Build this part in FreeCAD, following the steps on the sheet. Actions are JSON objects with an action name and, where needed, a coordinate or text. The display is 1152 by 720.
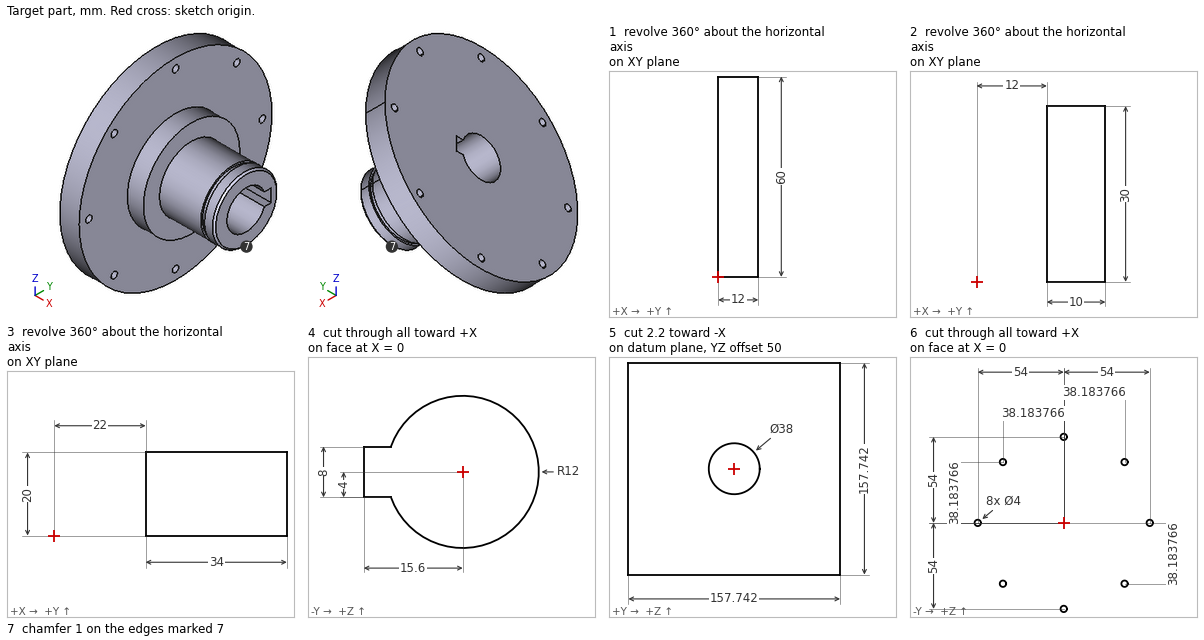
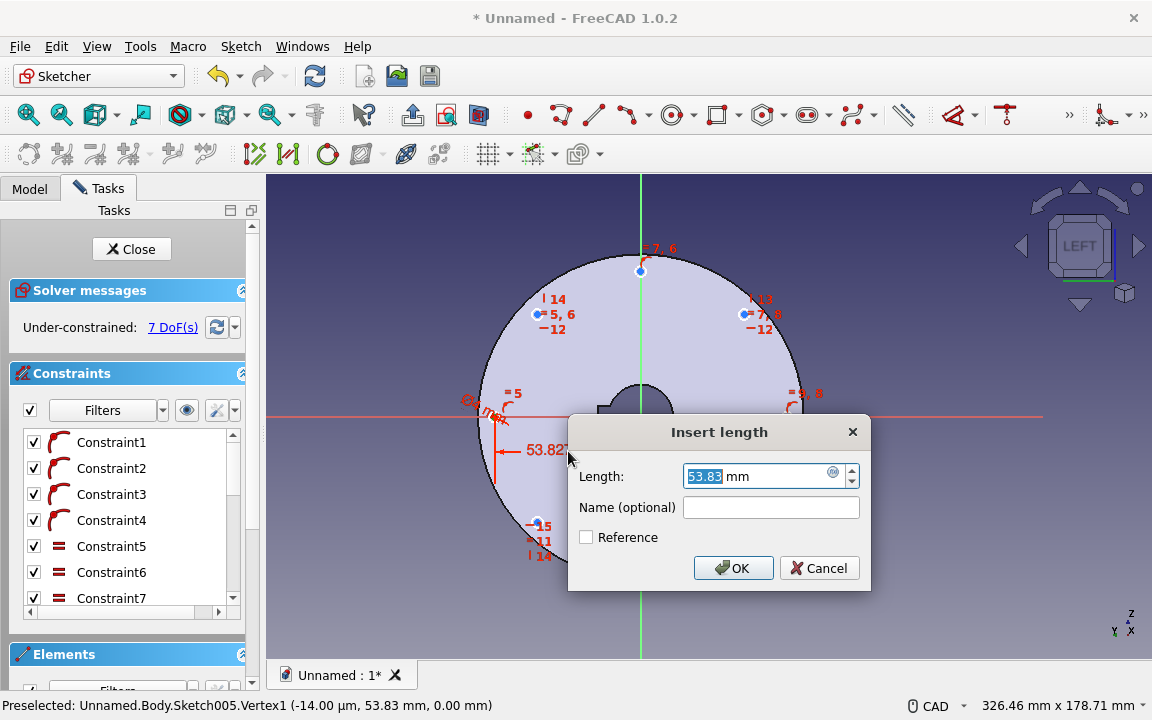
{"action": "type", "text": "54"}
{"action": "key", "text": "Return"}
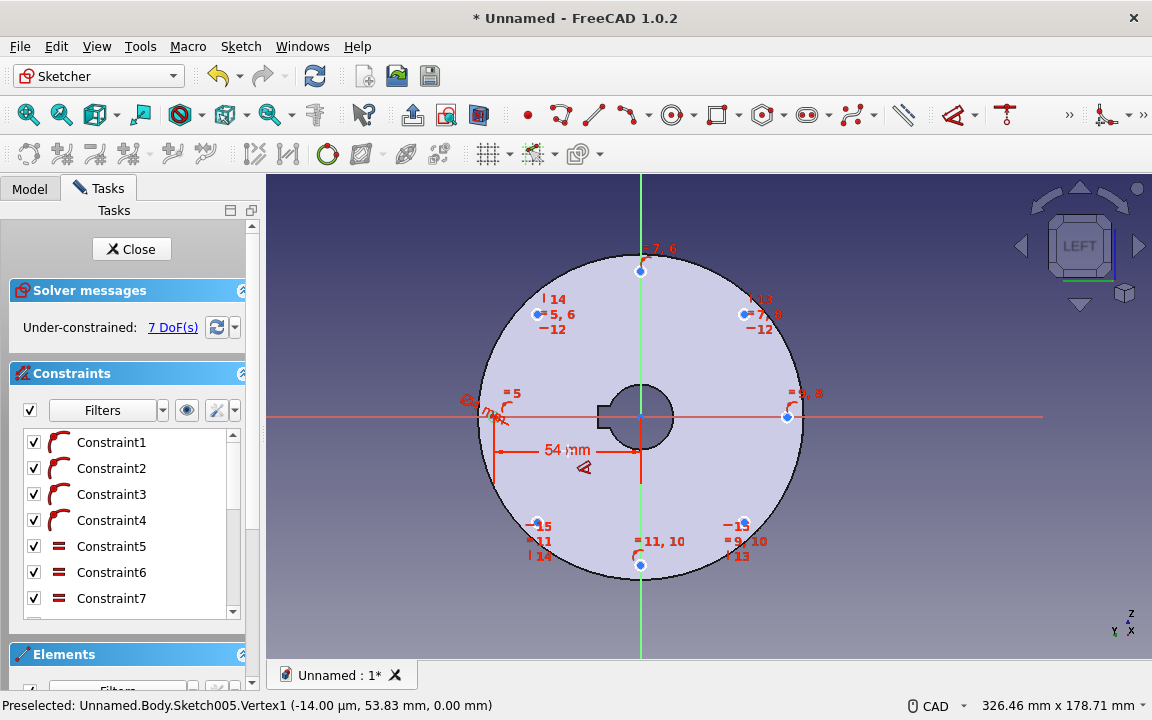
{"action": "left_click", "coordinate": [641, 272]}
{"action": "left_click", "coordinate": [675, 344]}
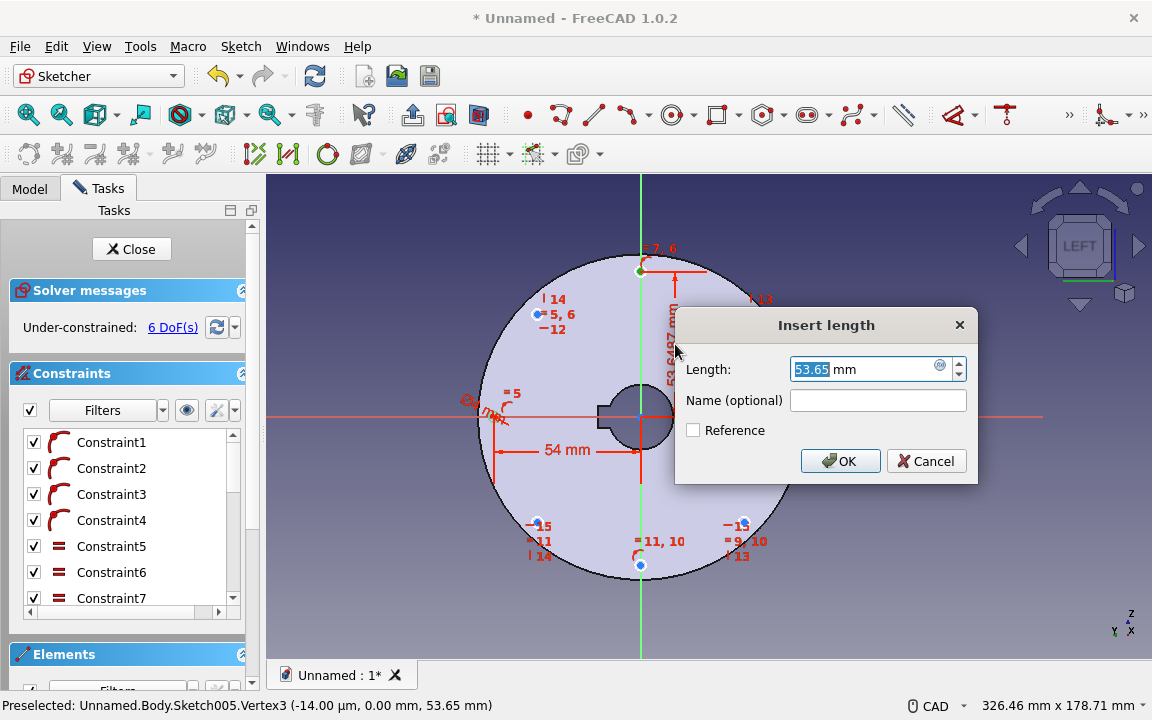
{"action": "type", "text": "54"}
{"action": "key", "text": "Return"}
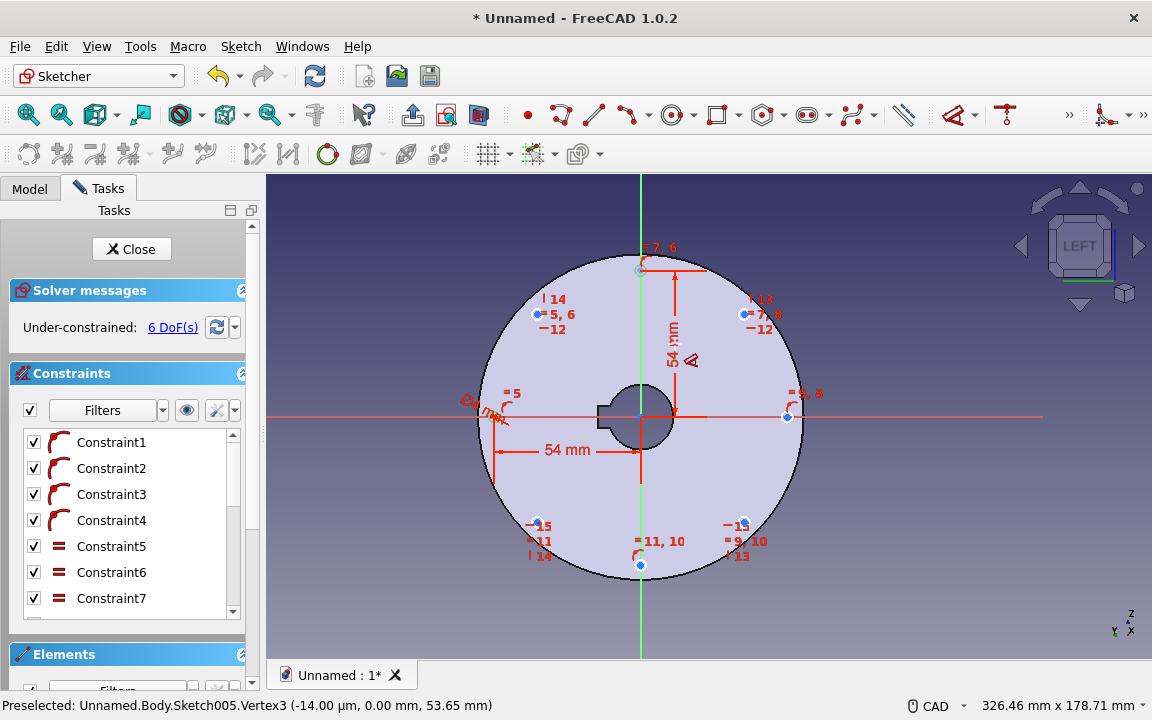
{"action": "left_click", "coordinate": [787, 417]}
{"action": "left_click", "coordinate": [714, 451]}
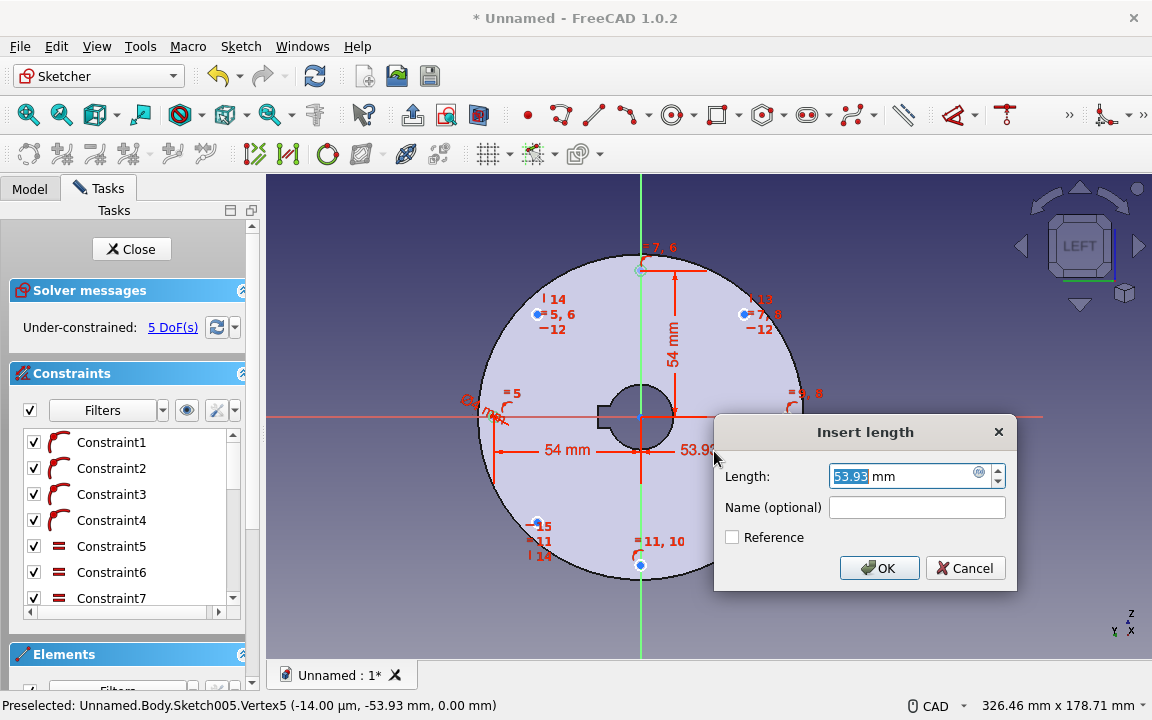
{"action": "type", "text": "54"}
{"action": "key", "text": "Return"}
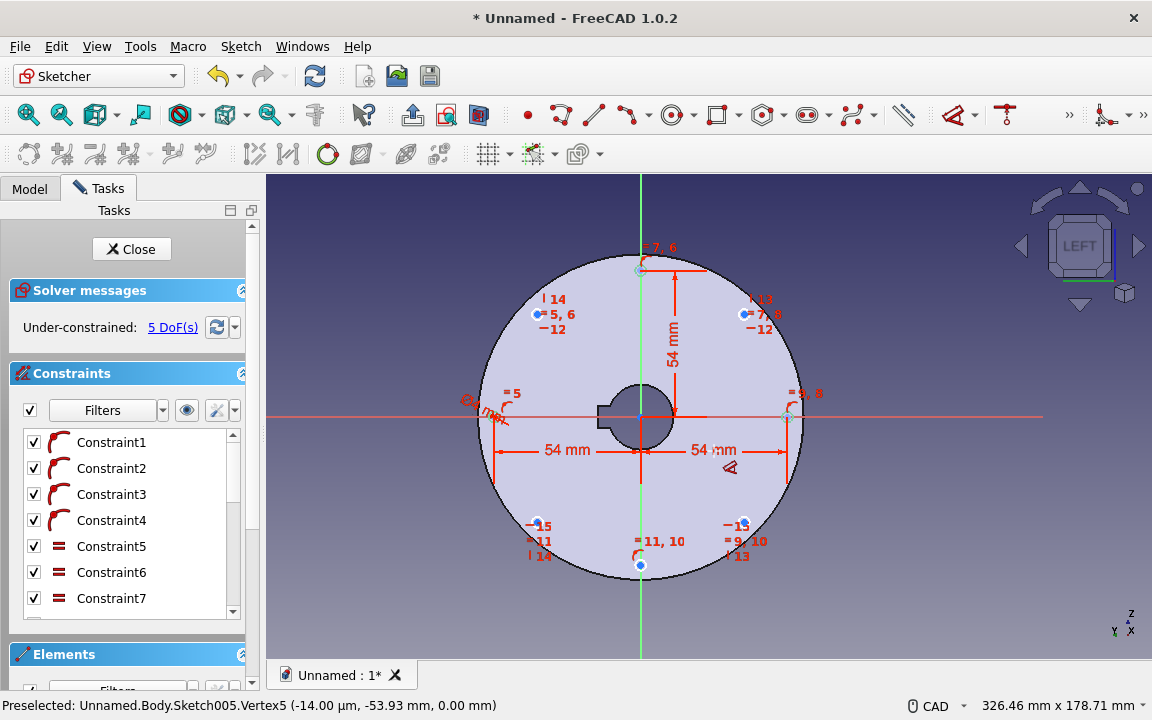
{"action": "left_click", "coordinate": [641, 565]}
{"action": "left_click", "coordinate": [675, 491]}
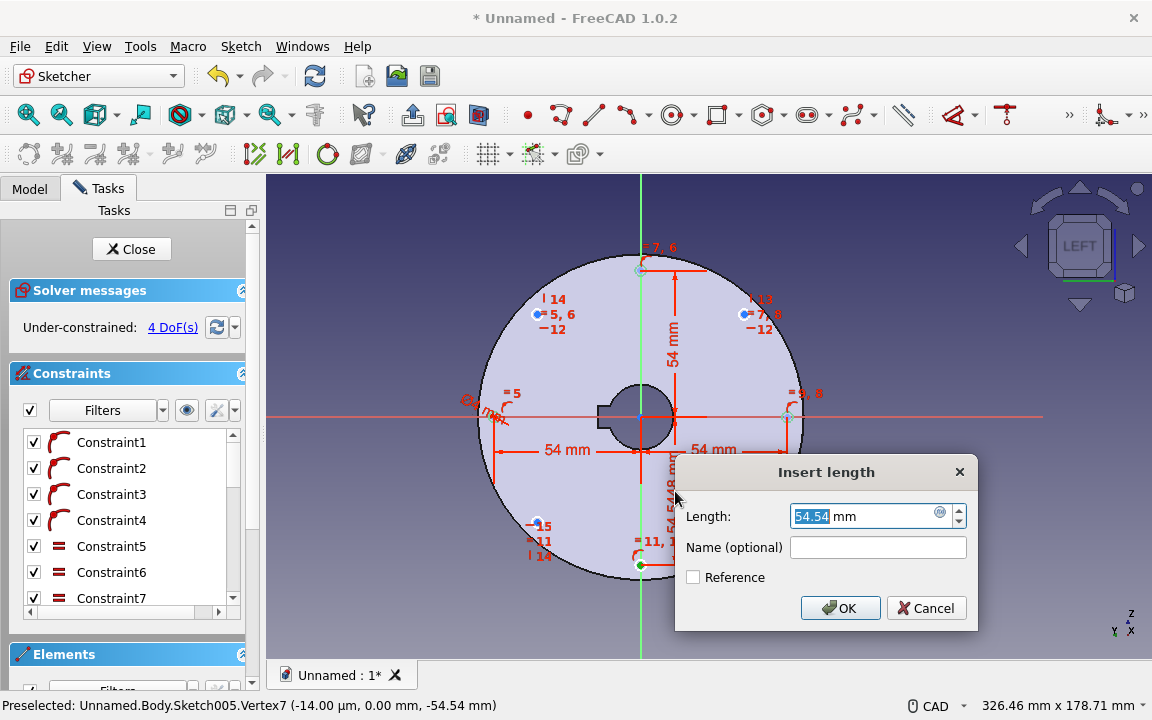
{"action": "type", "text": "54"}
{"action": "key", "text": "Return"}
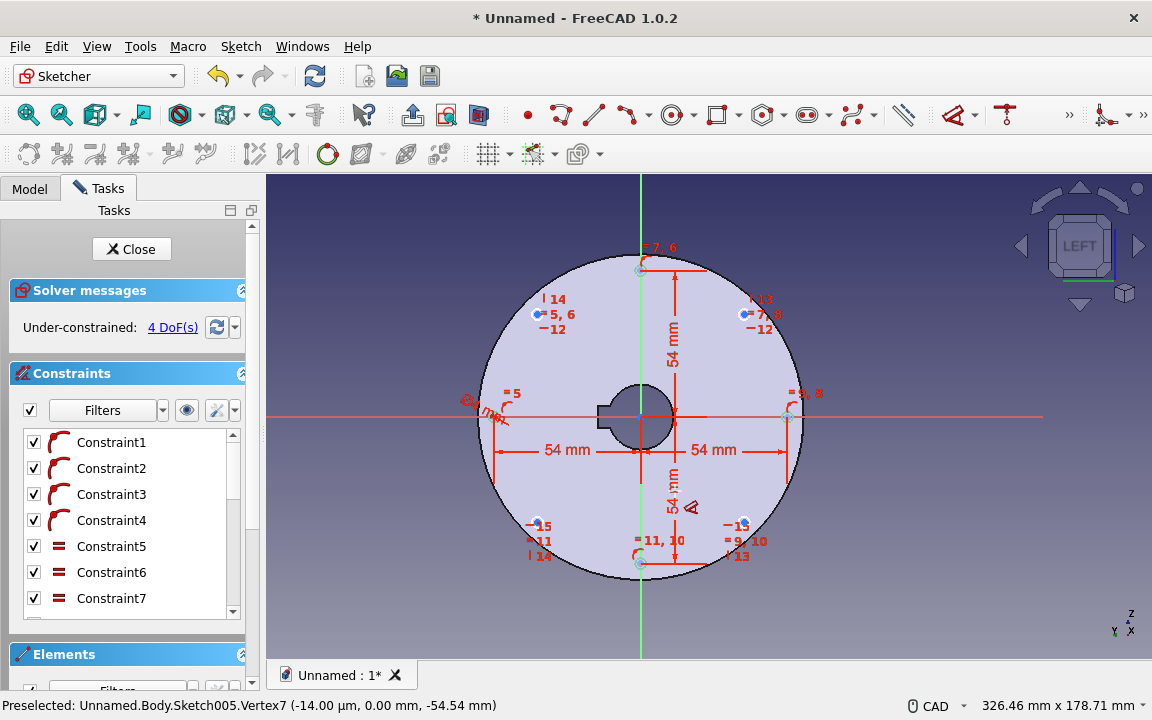
{"action": "left_click", "coordinate": [537, 315]}
{"action": "left_click", "coordinate": [589, 281]}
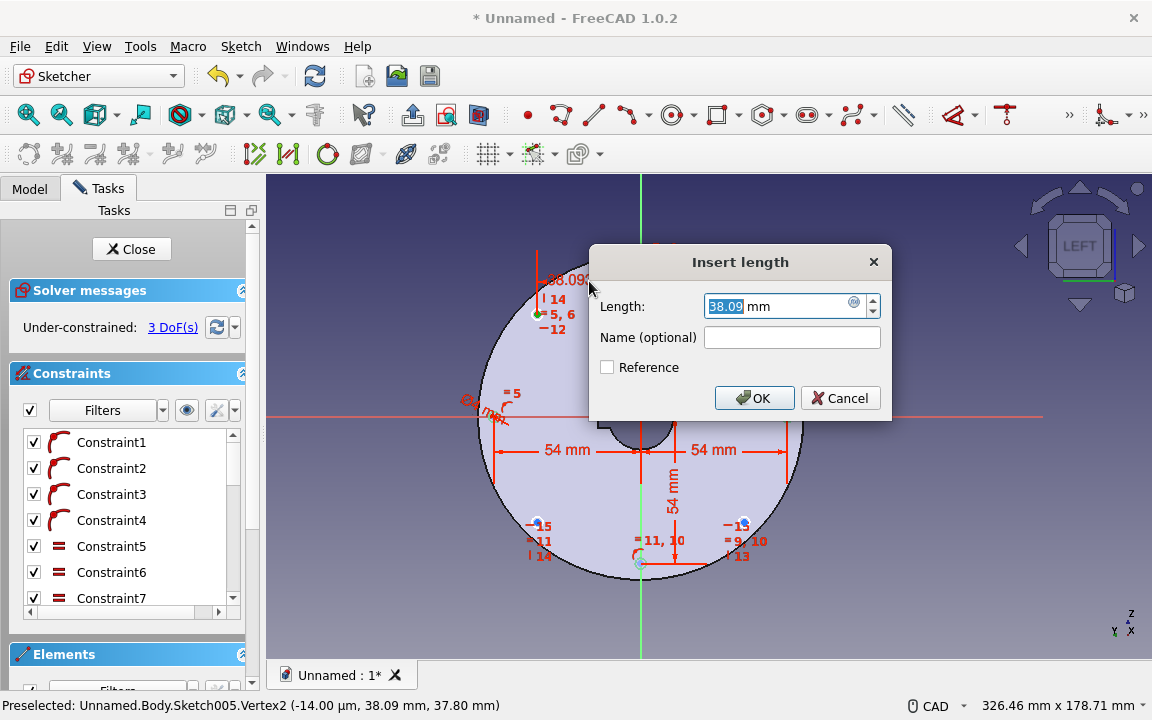
{"action": "type", "text": "38.183766"}
{"action": "key", "text": "Return"}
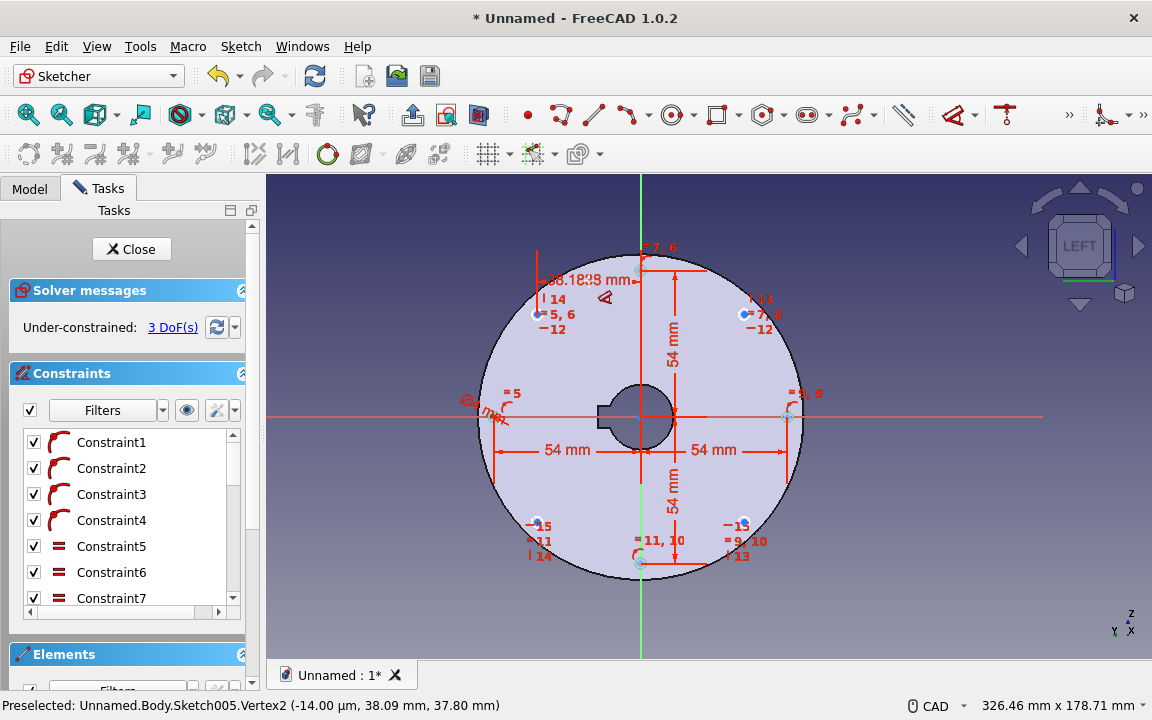
{"action": "left_click", "coordinate": [537, 315]}
{"action": "left_click", "coordinate": [503, 366]}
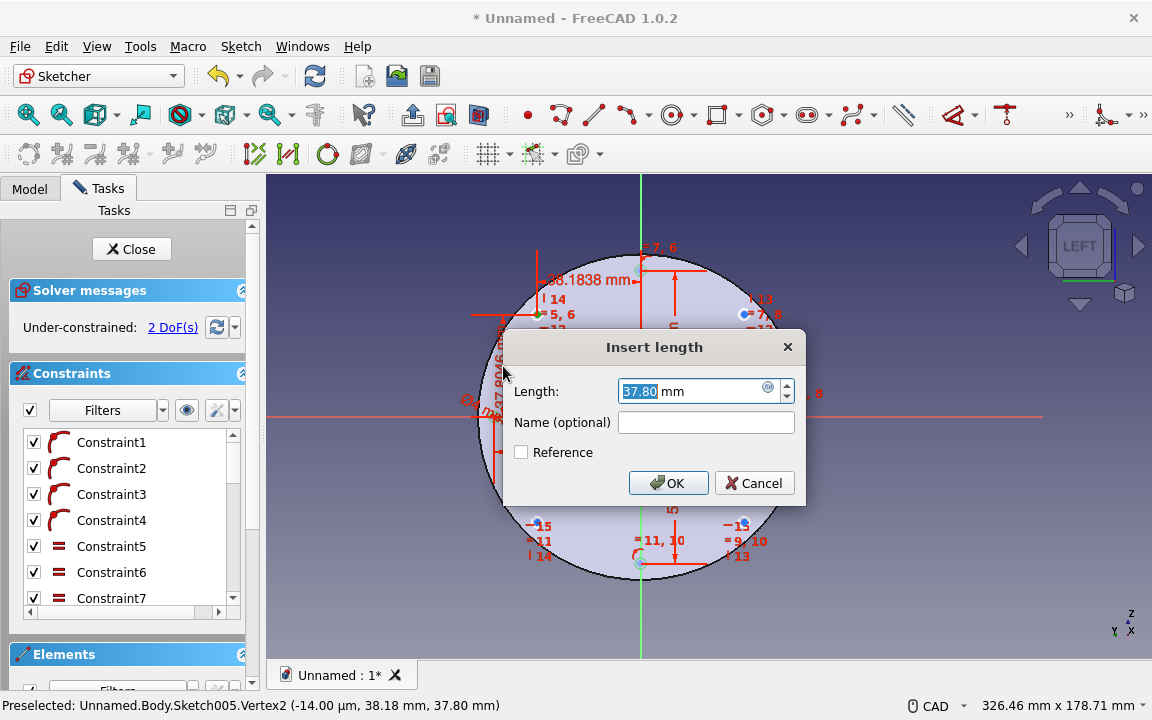
{"action": "type", "text": "38.183766"}
{"action": "key", "text": "Return"}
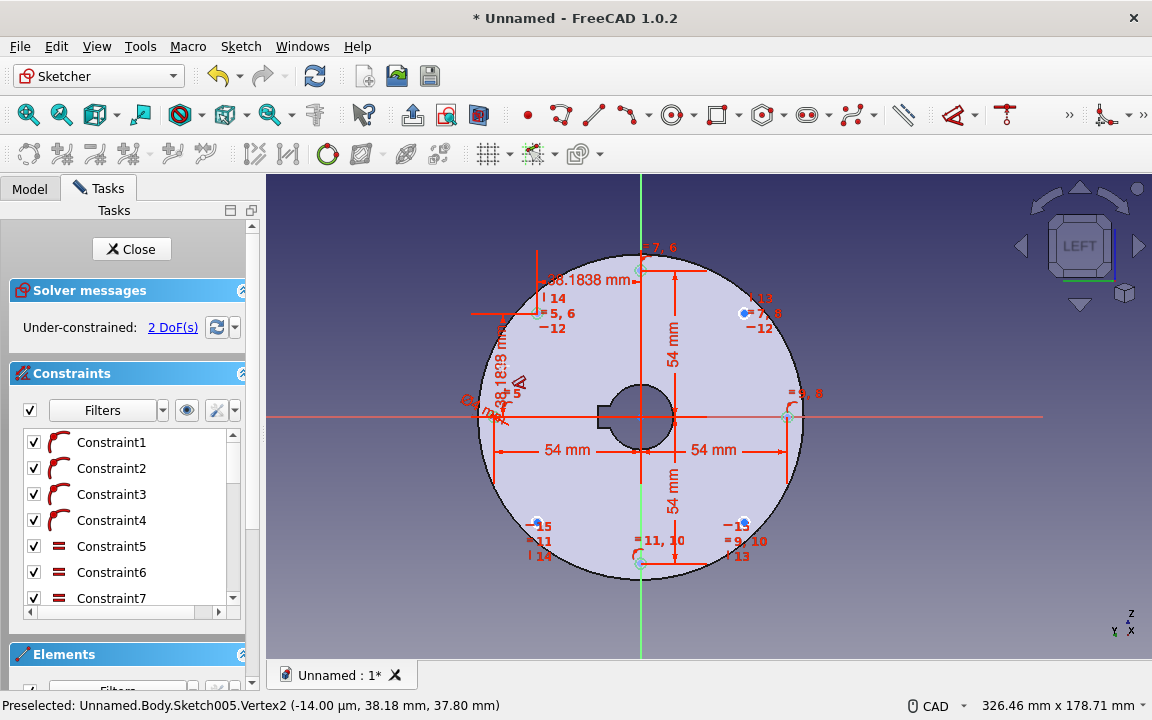
{"action": "left_click", "coordinate": [744, 314]}
{"action": "left_click", "coordinate": [692, 280]}